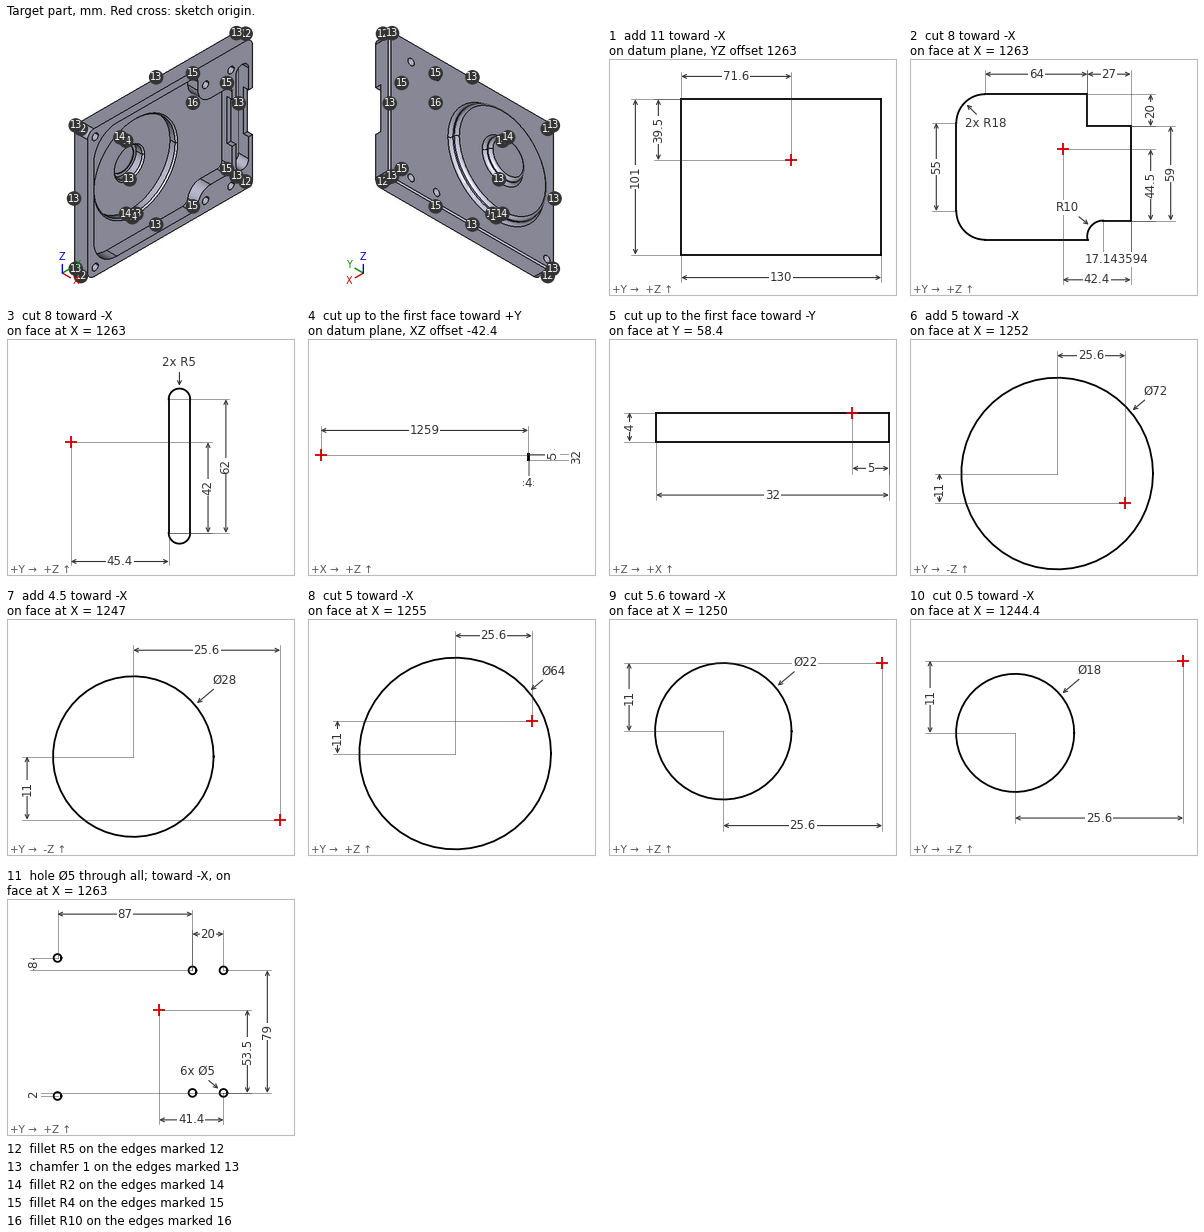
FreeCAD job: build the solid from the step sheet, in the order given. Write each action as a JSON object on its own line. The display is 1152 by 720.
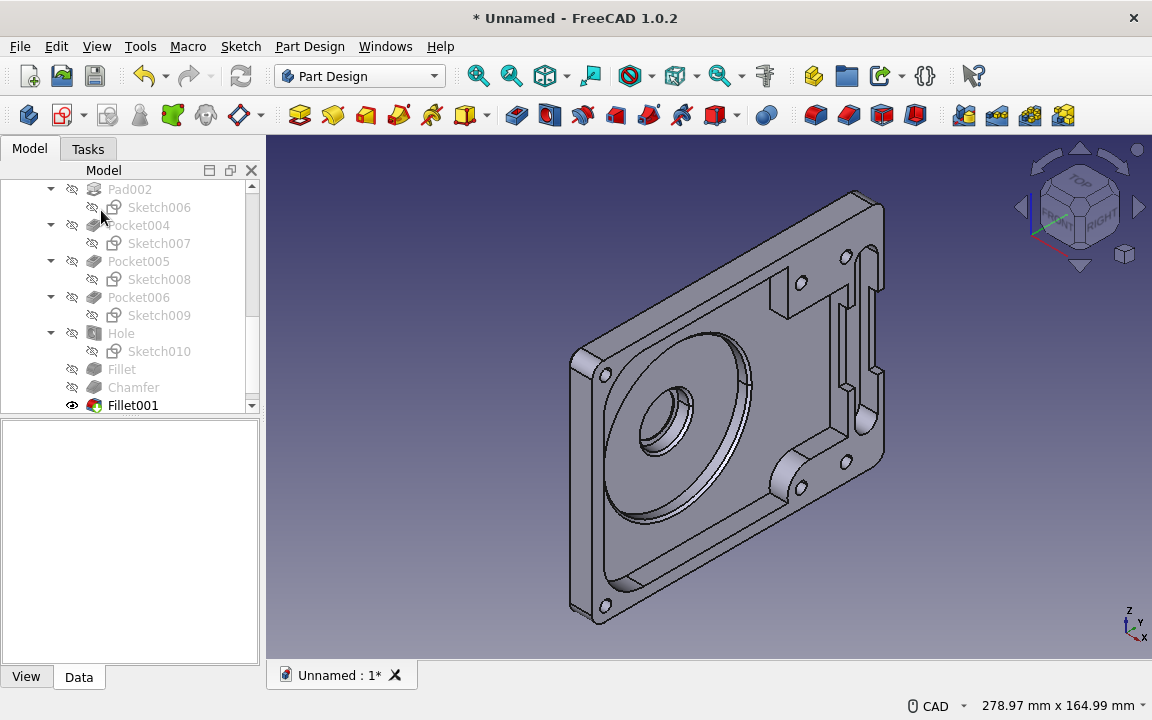
{"action": "key", "text": "1"}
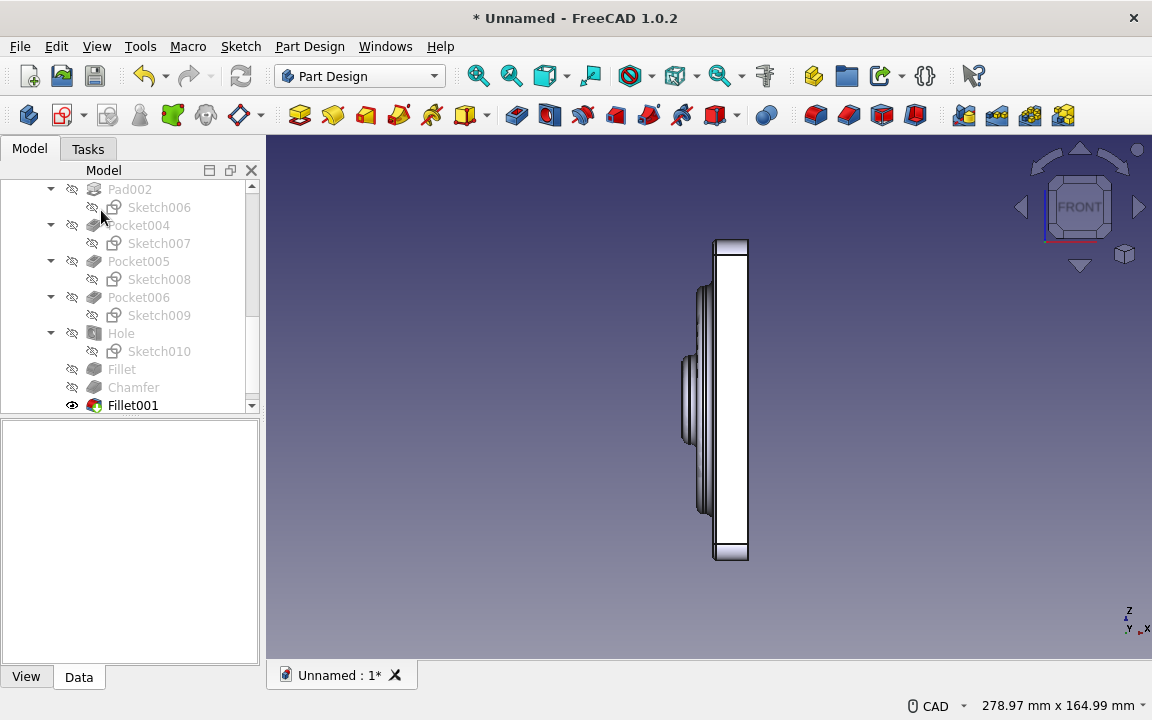
{"action": "key", "text": "3"}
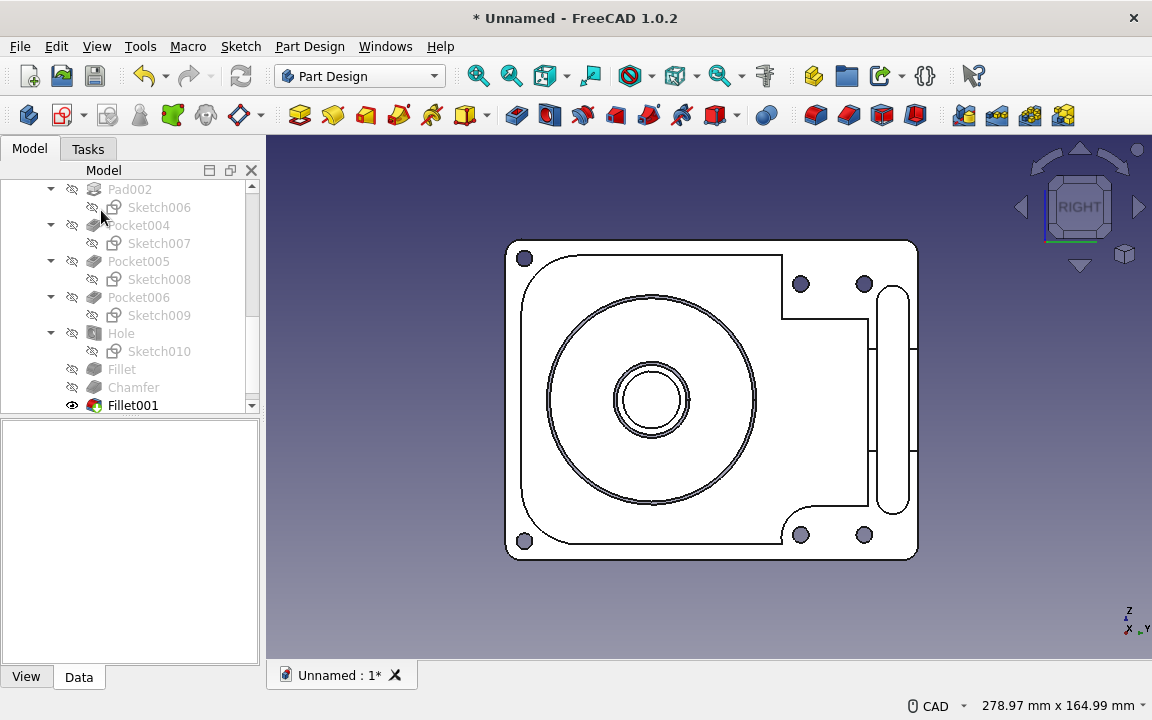
{"action": "key", "text": "5"}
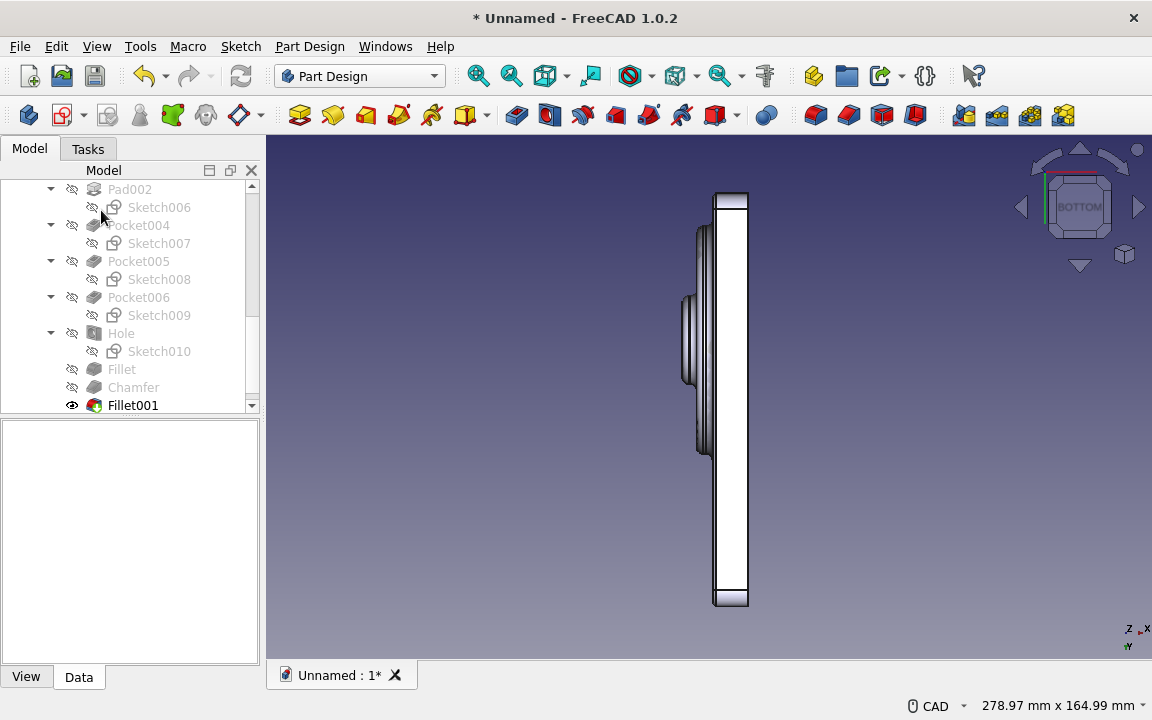
{"action": "key", "text": "4"}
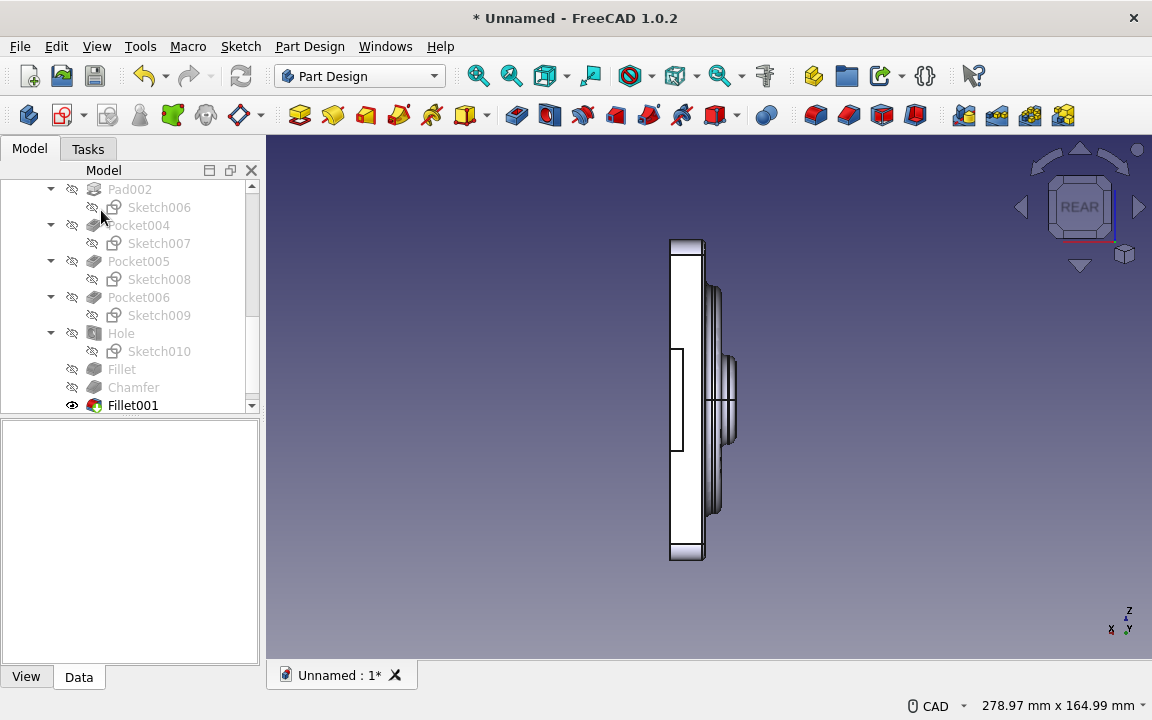
{"action": "key", "text": "6"}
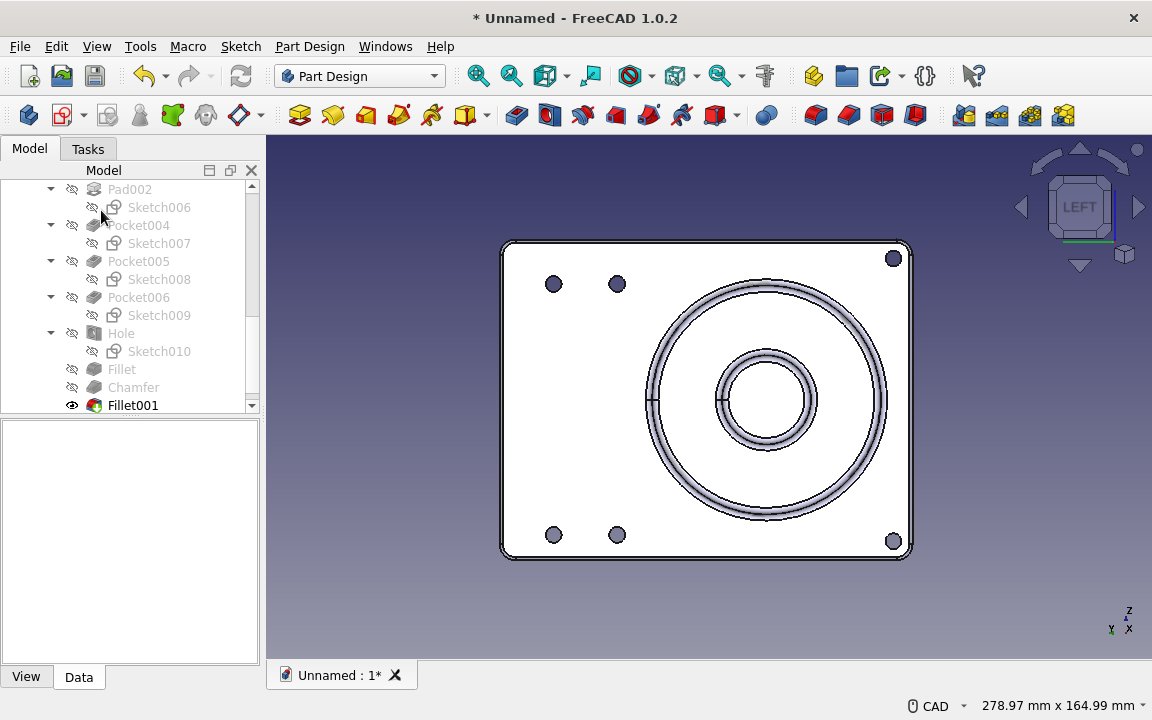
{"action": "key", "text": "v 3"}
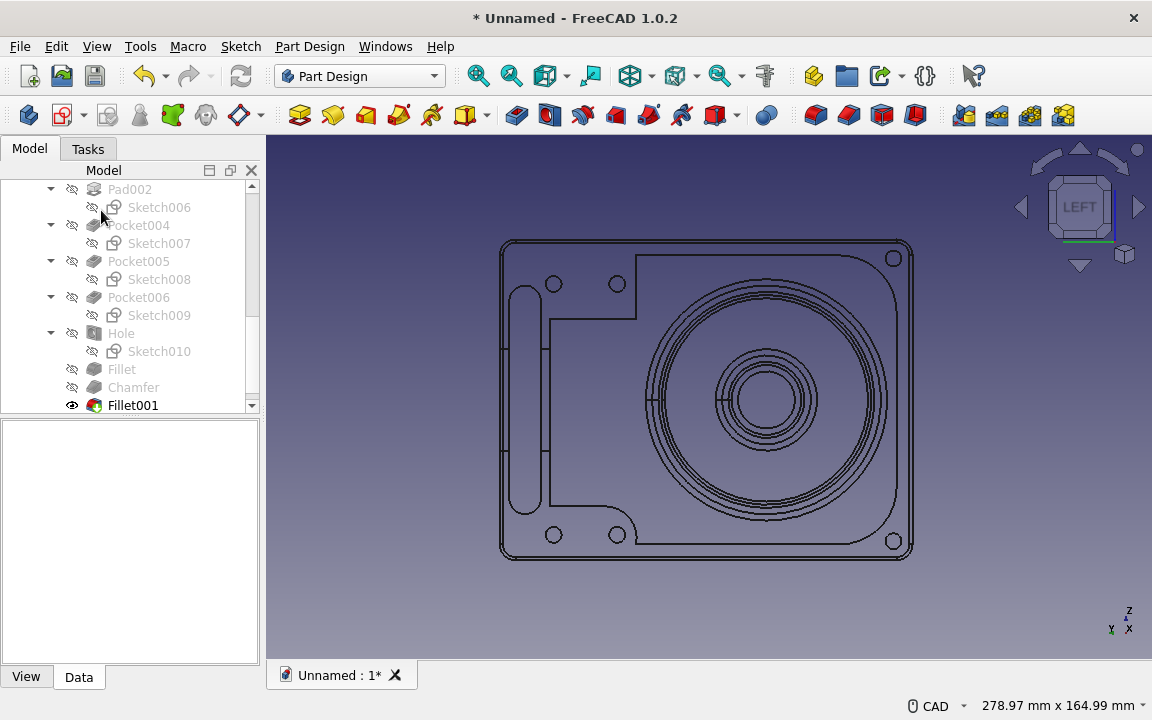
{"action": "key", "text": "0"}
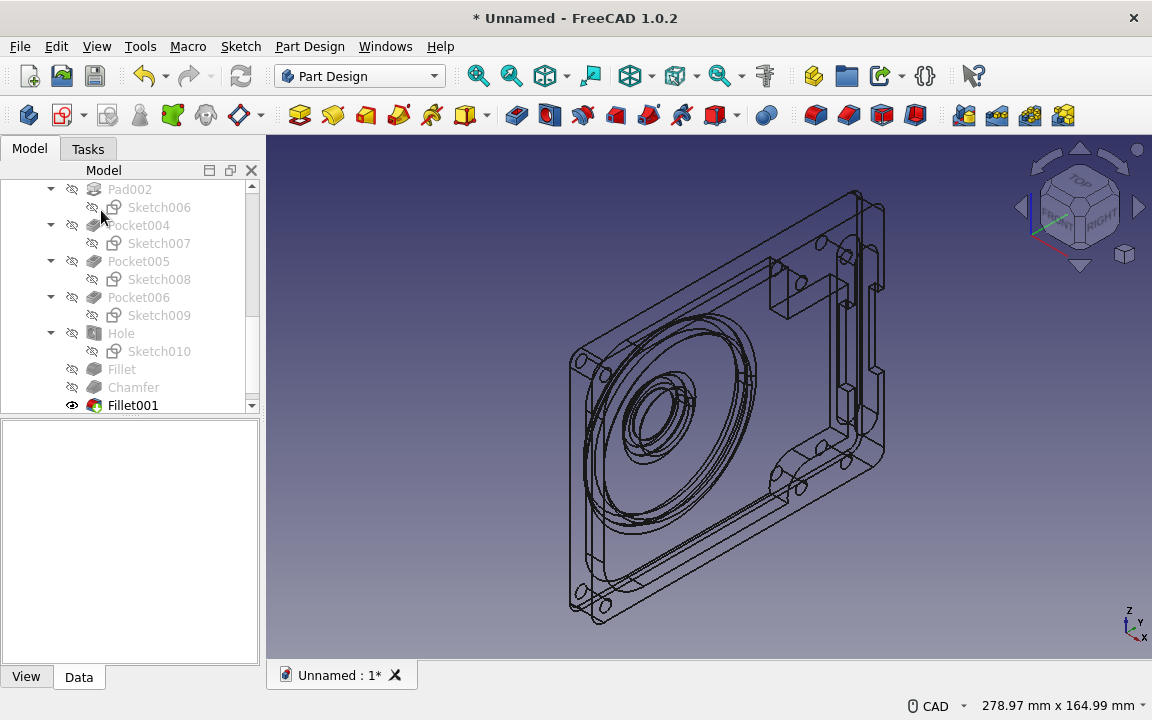
{"action": "left_click", "coordinate": [779, 497]}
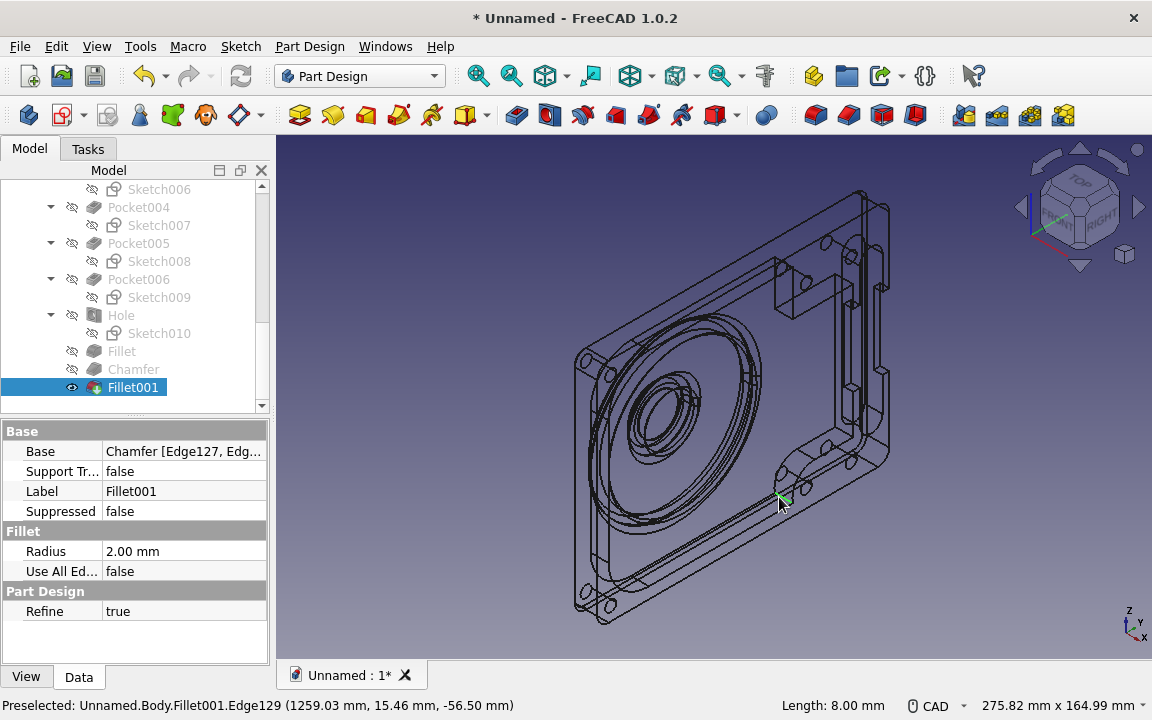
{"action": "left_click", "coordinate": [844, 278], "text": "ctrl"}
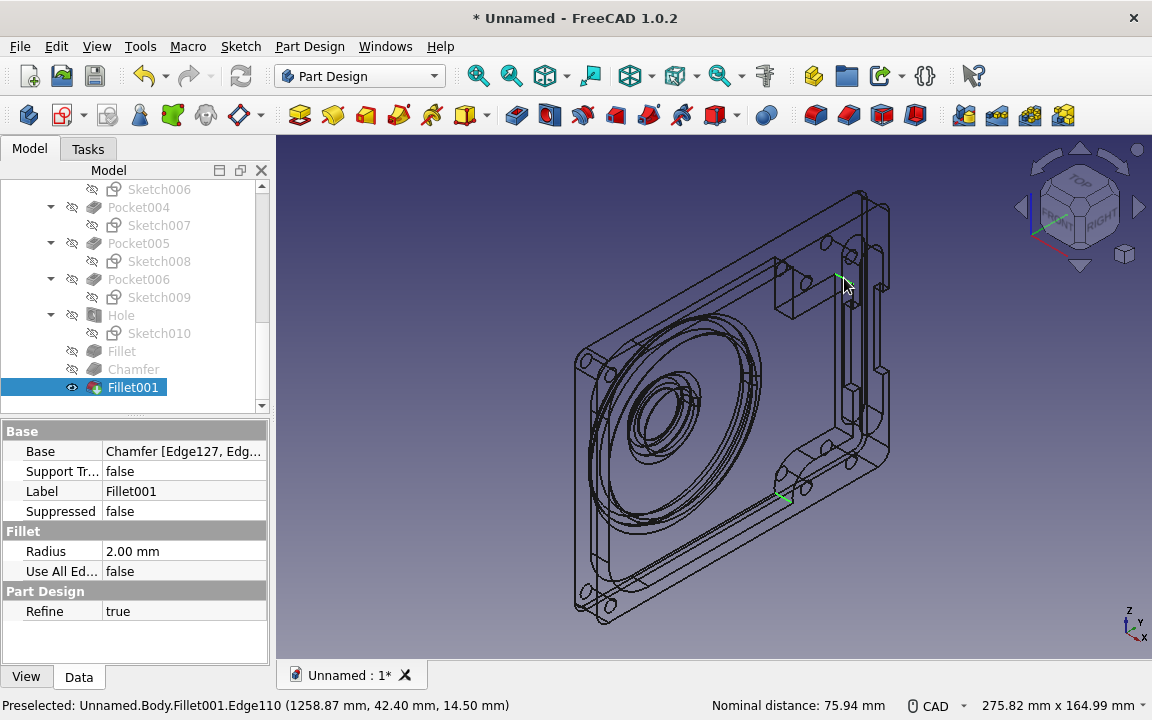
{"action": "left_click", "coordinate": [844, 431], "text": "ctrl"}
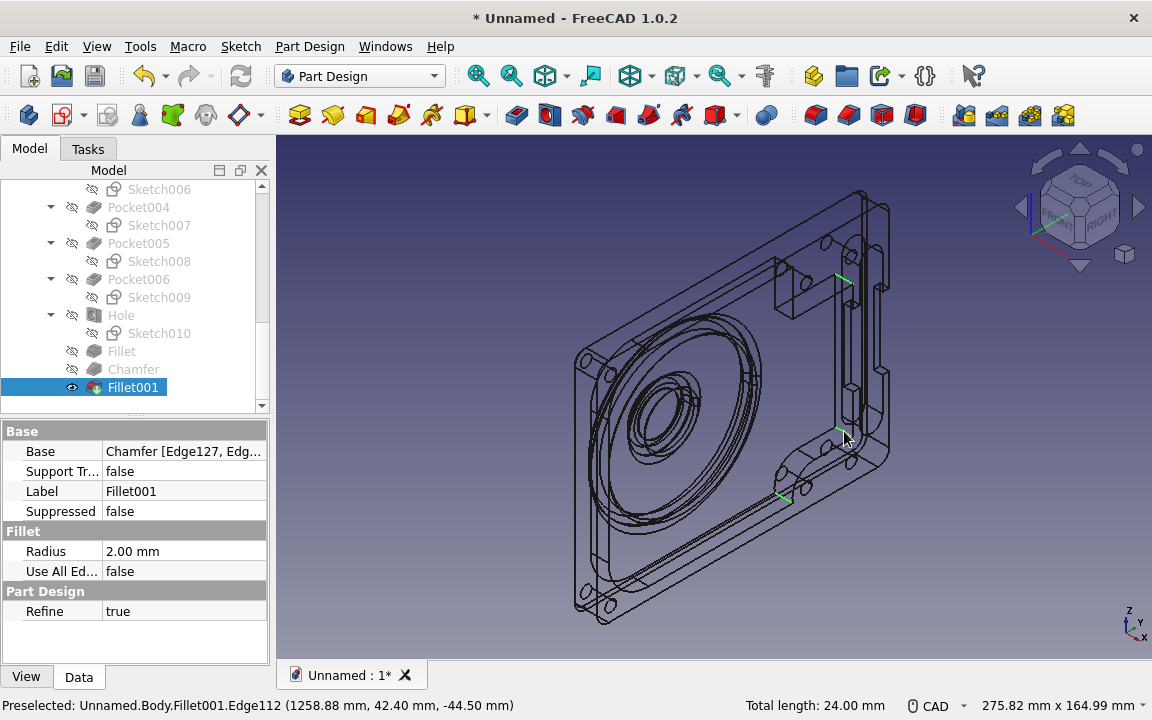
{"action": "scroll", "coordinate": [784, 261], "scroll_direction": "up", "scroll_amount": 6}